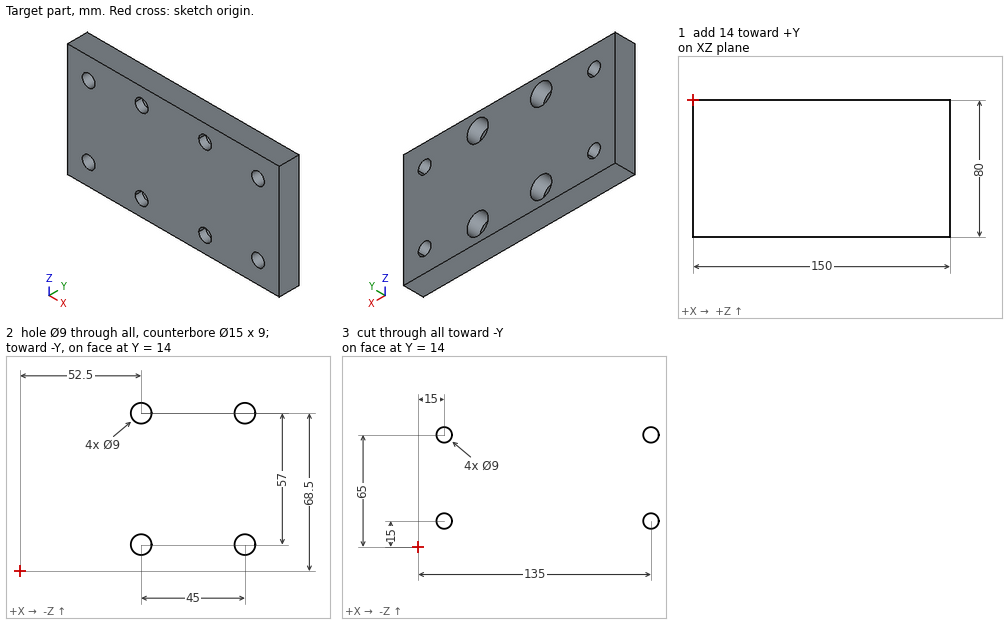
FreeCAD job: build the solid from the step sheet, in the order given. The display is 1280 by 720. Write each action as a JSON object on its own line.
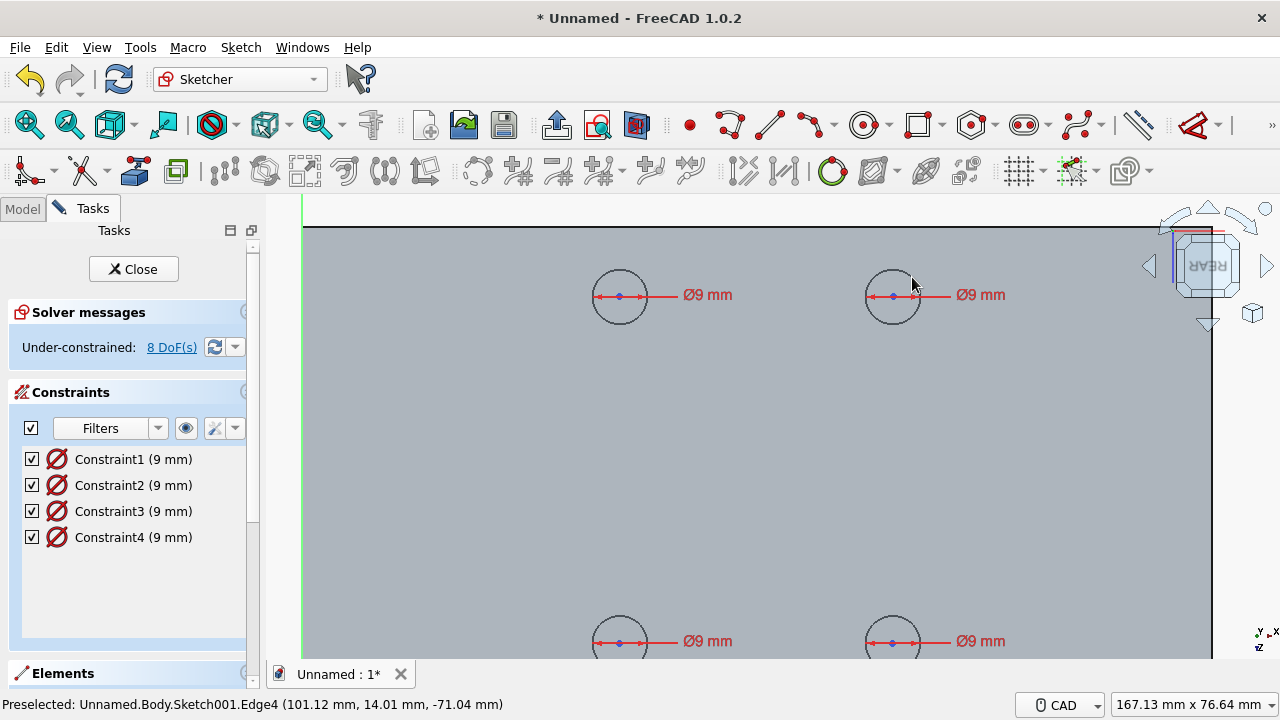
{"action": "left_click", "coordinate": [620, 297]}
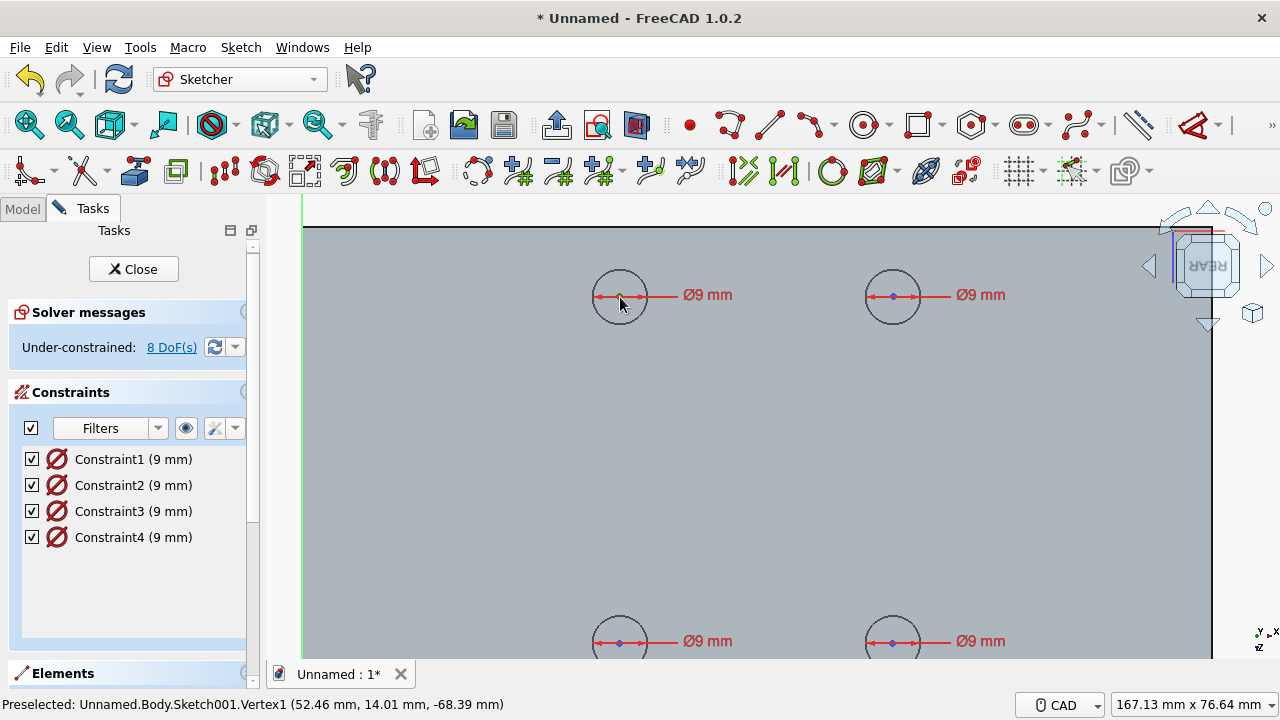
{"action": "scroll", "coordinate": [895, 296], "scroll_direction": "down", "scroll_amount": 2}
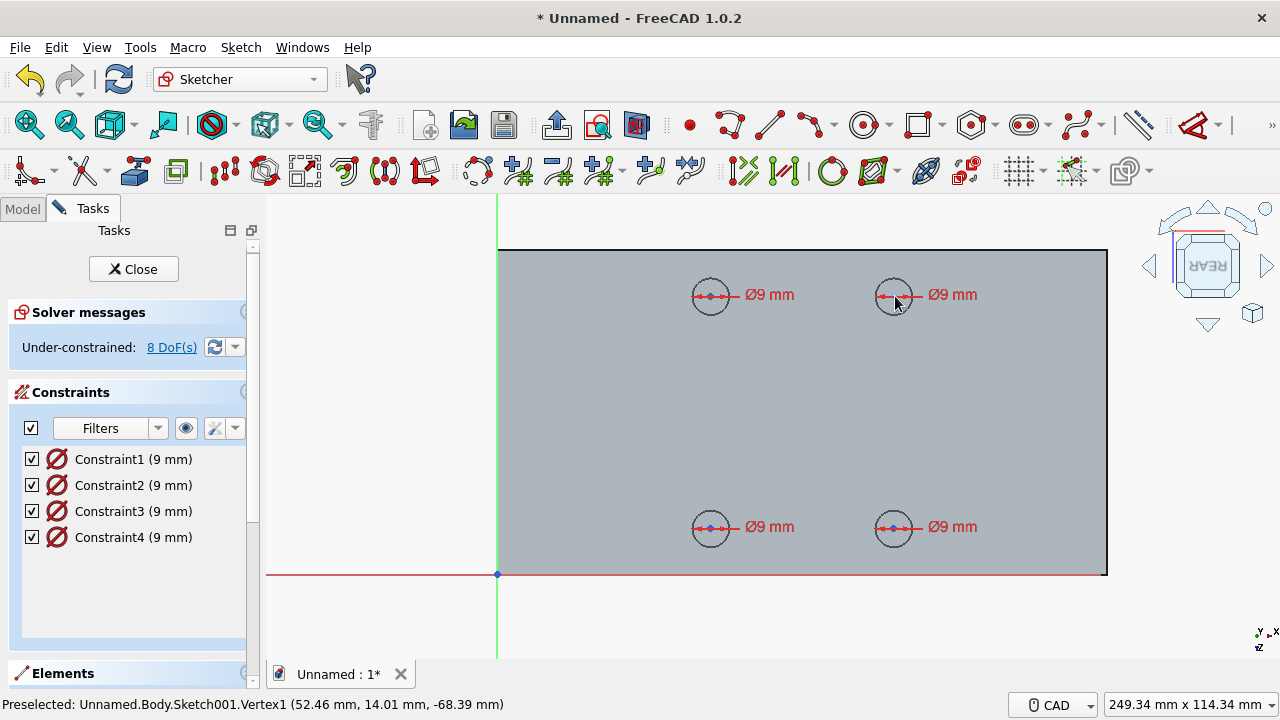
{"action": "left_click", "coordinate": [711, 529]}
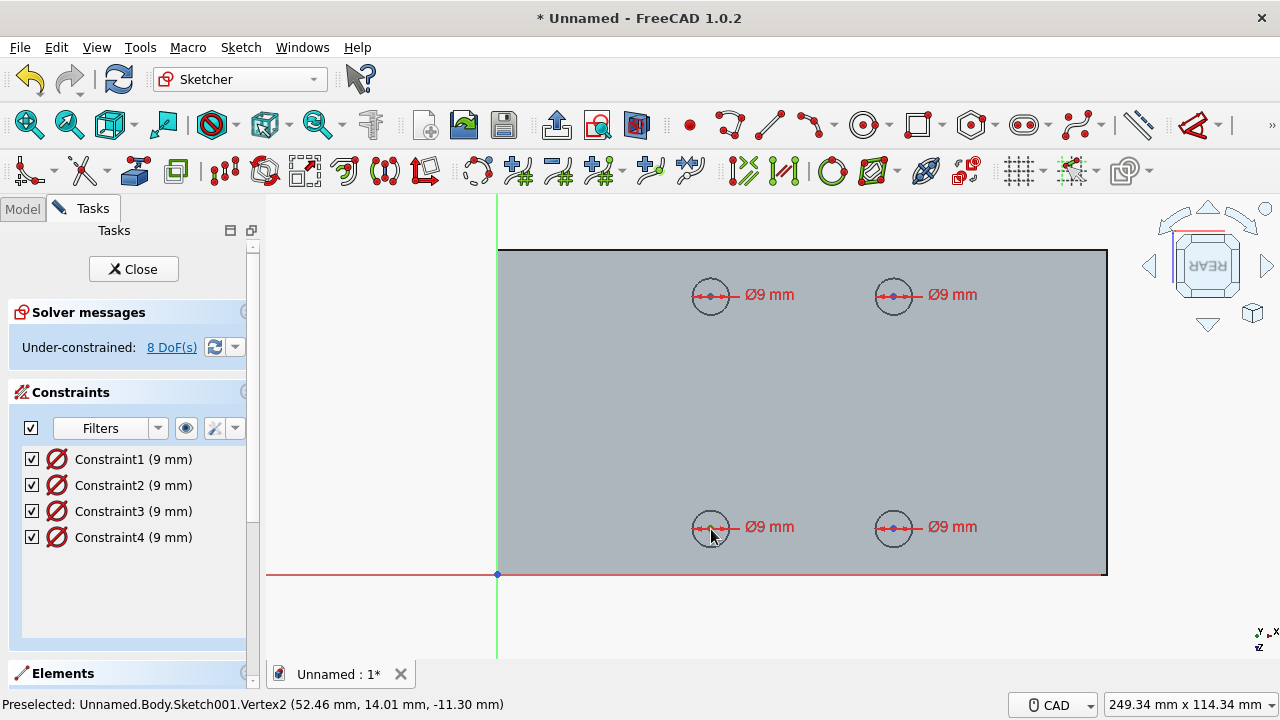
{"action": "key", "text": "v"}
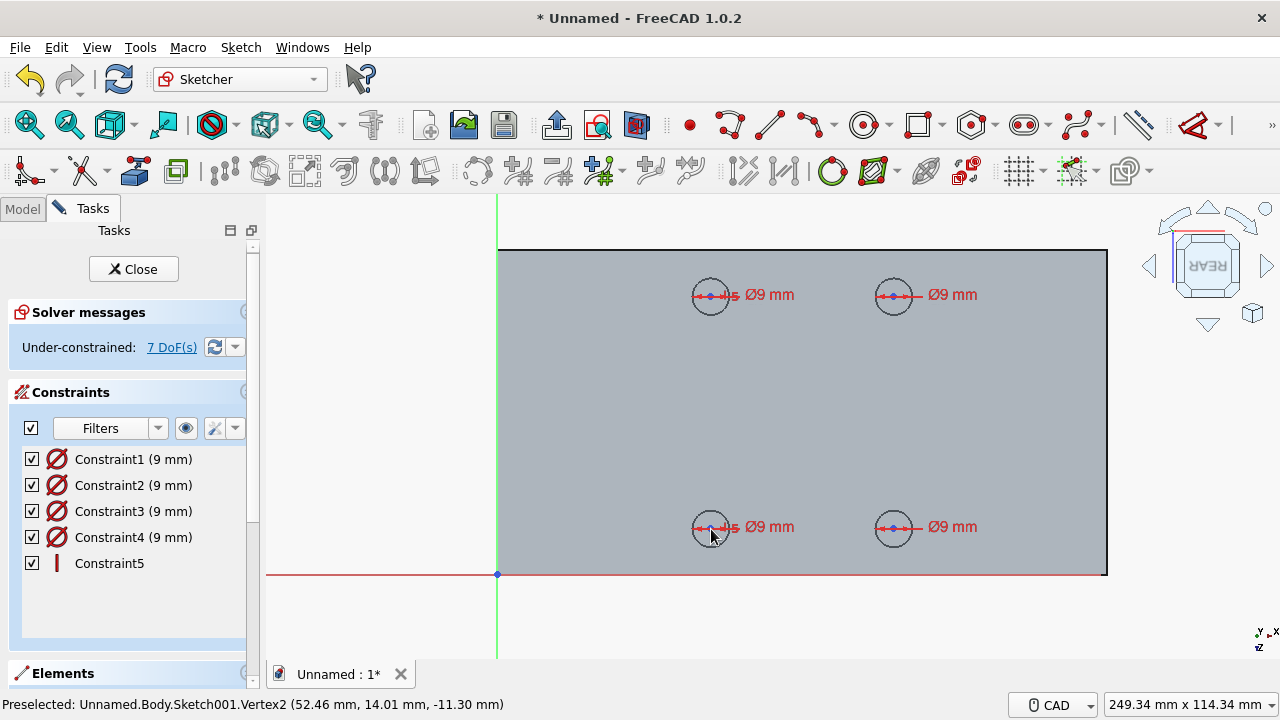
{"action": "left_click", "coordinate": [711, 529]}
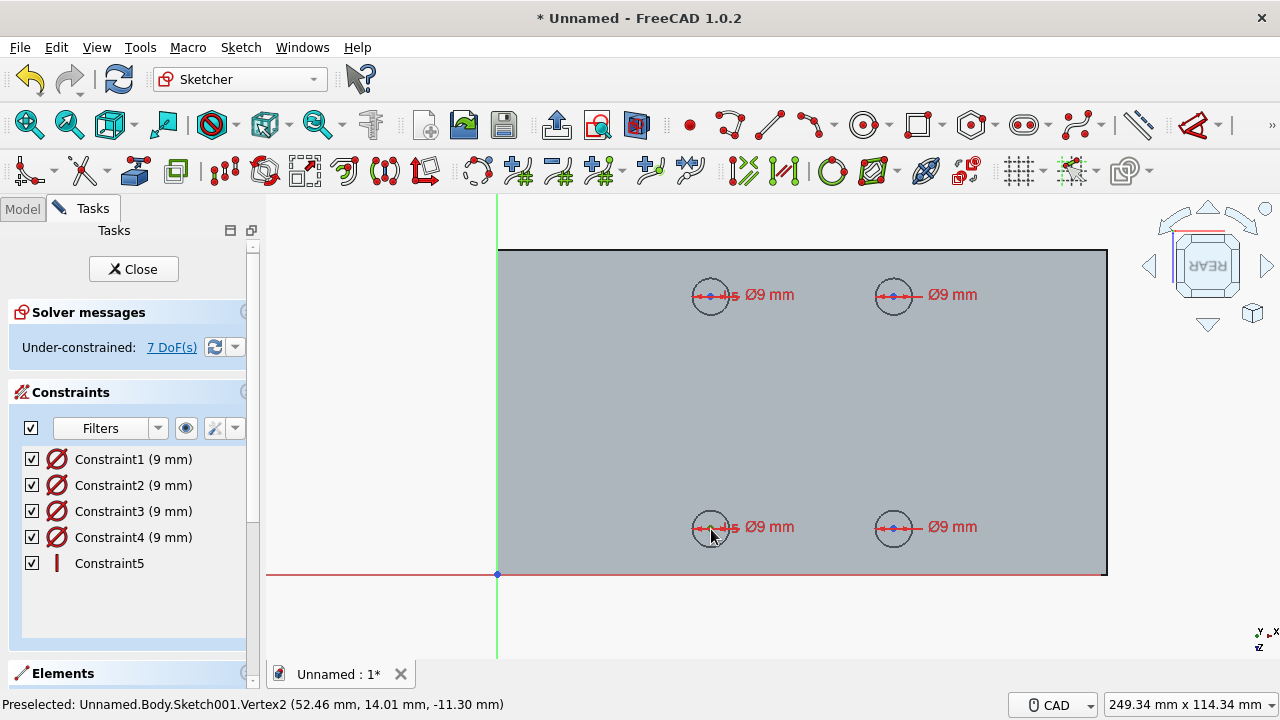
{"action": "left_click", "coordinate": [894, 529]}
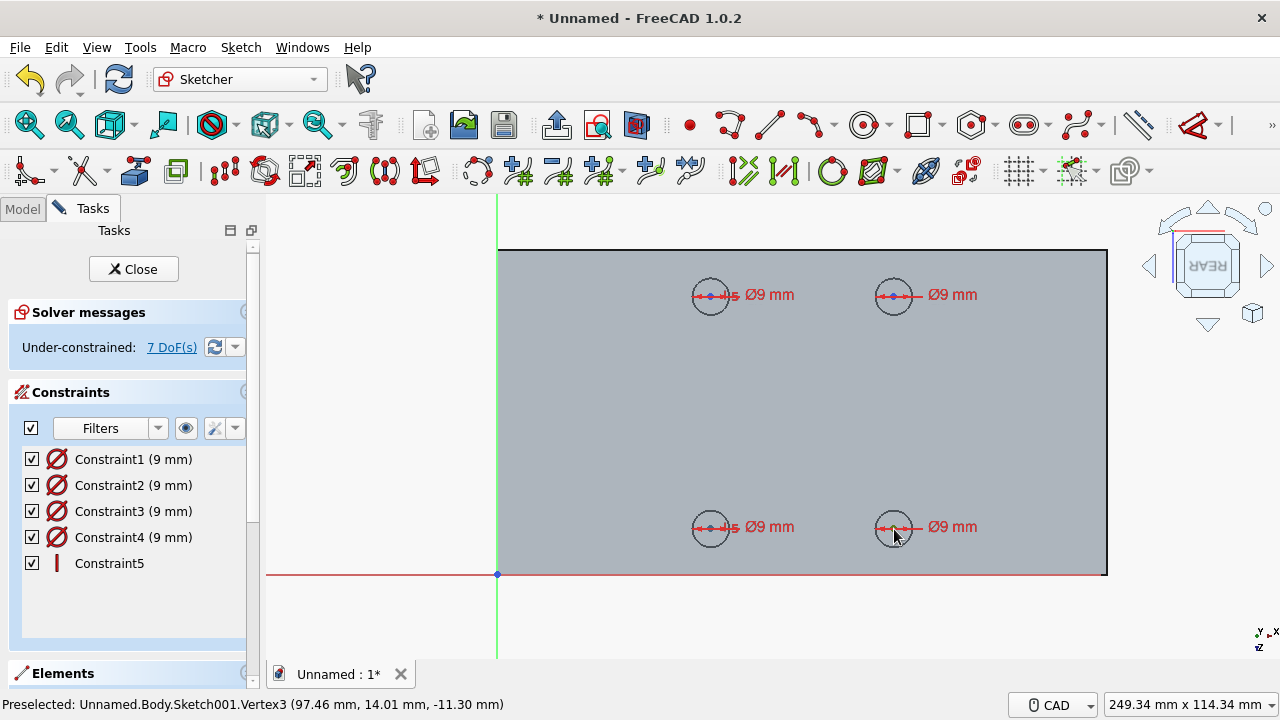
{"action": "key", "text": "h"}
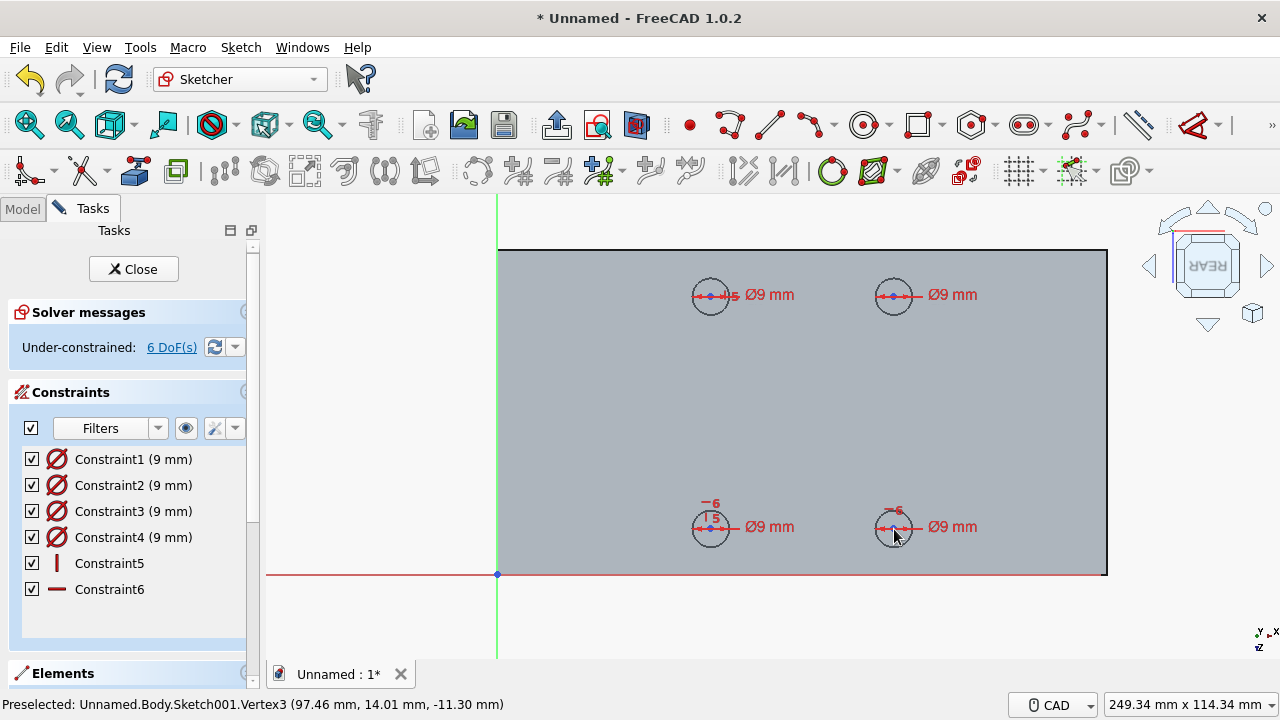
{"action": "left_click", "coordinate": [894, 529]}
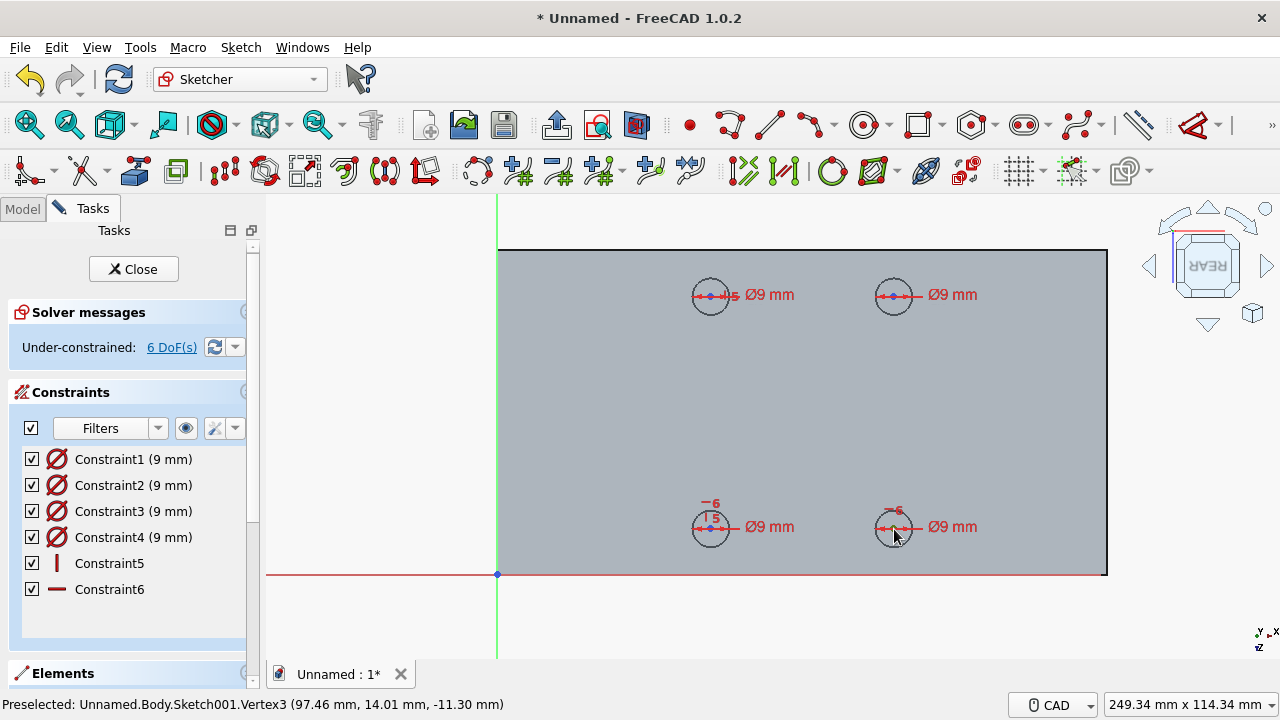
{"action": "left_click", "coordinate": [894, 297]}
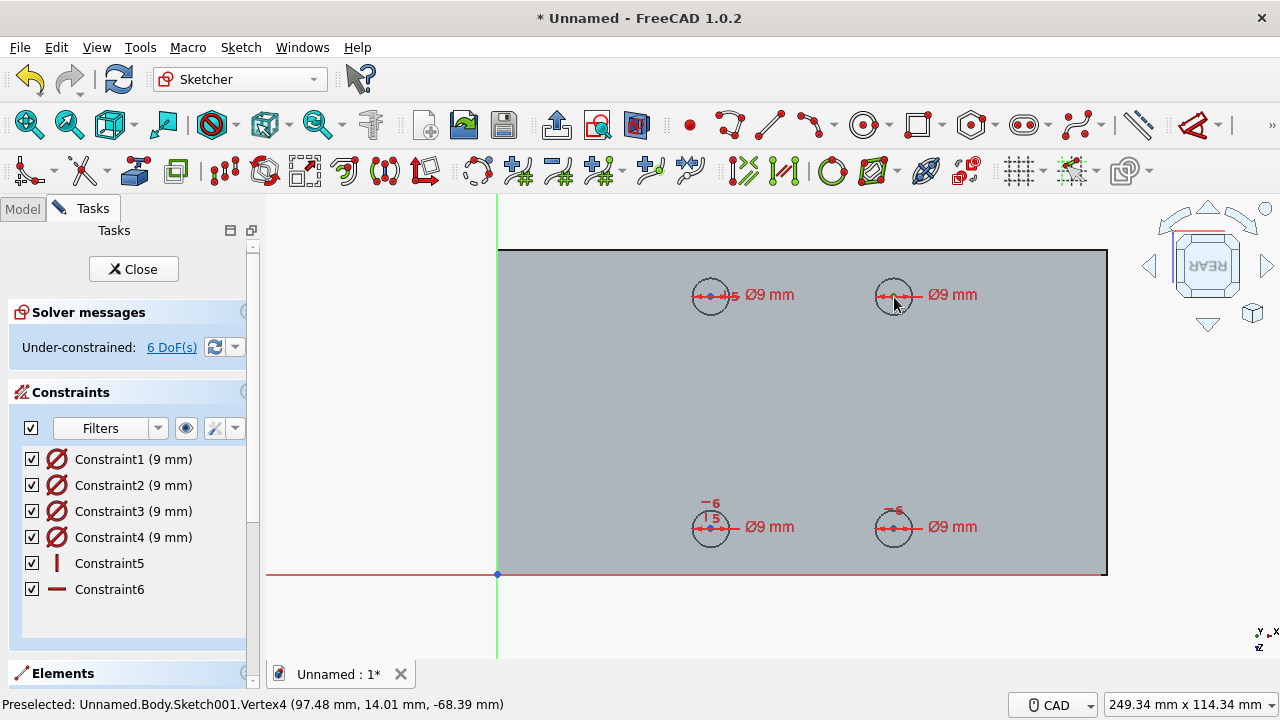
{"action": "key", "text": "v"}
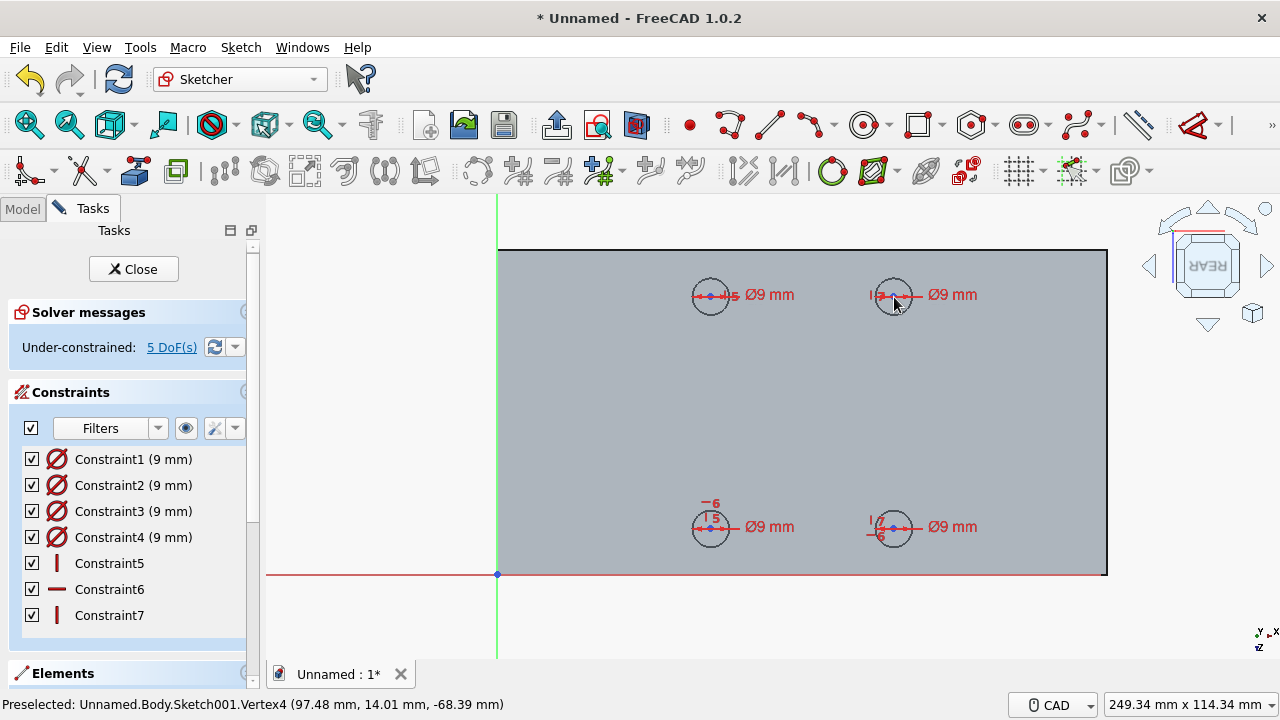
{"action": "left_click", "coordinate": [711, 297]}